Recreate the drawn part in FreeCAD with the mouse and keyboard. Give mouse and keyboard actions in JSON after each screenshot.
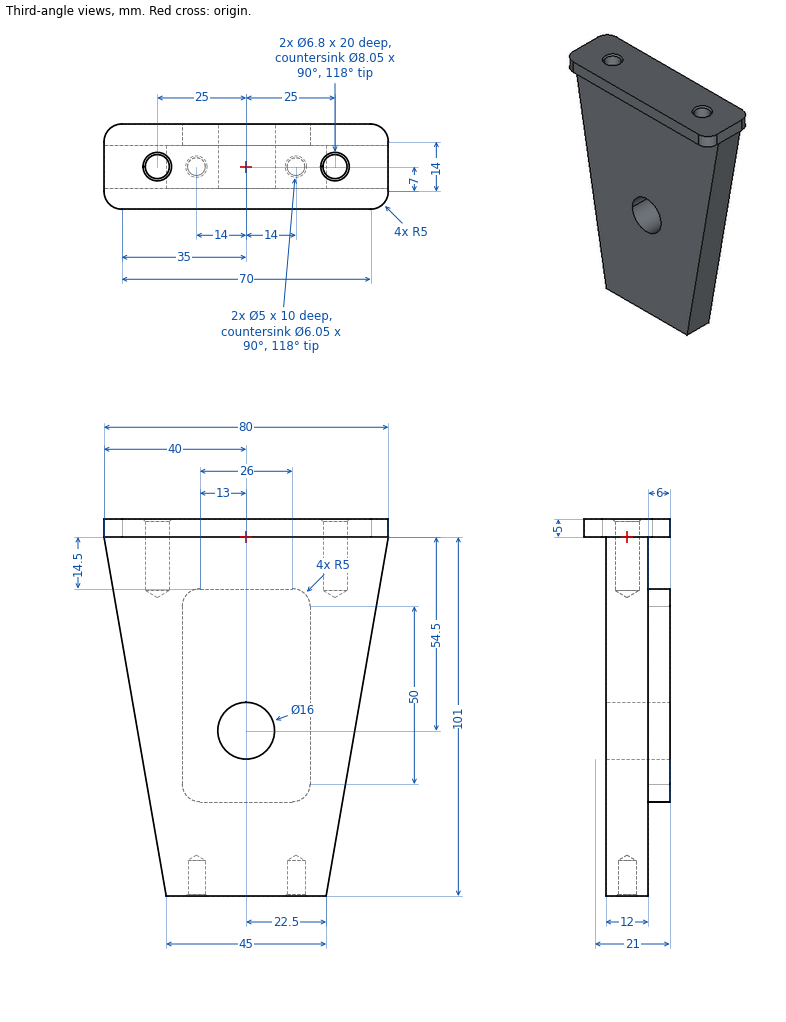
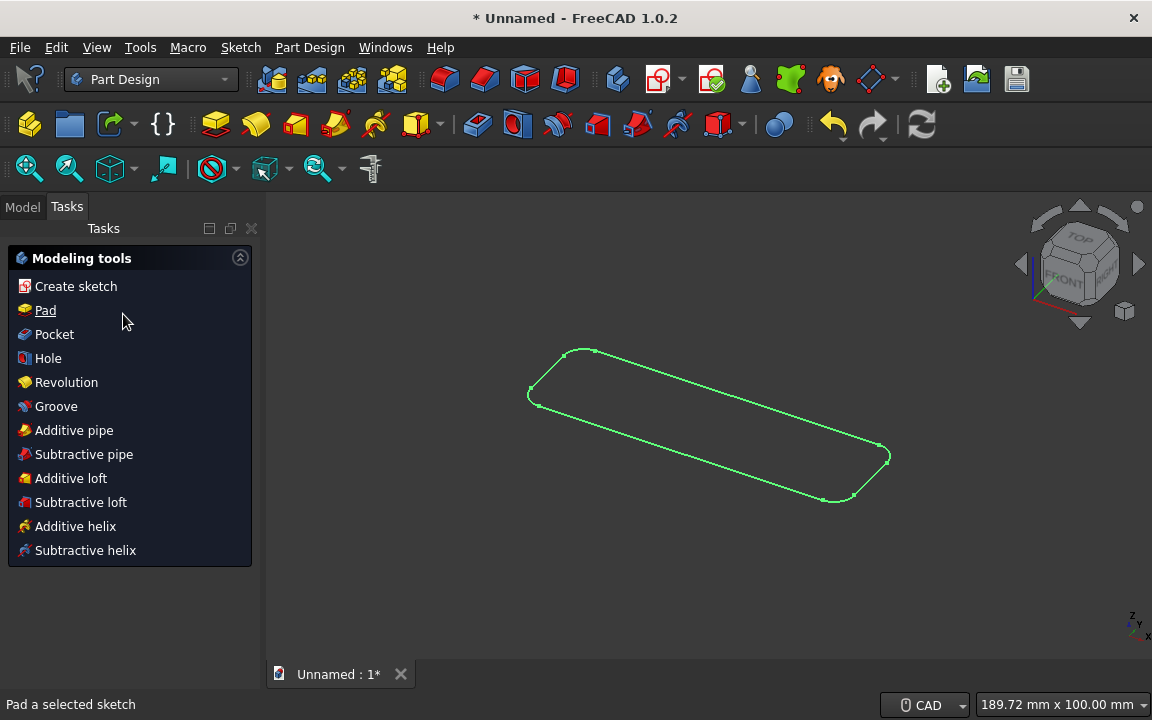
{"action": "left_click", "coordinate": [216, 124]}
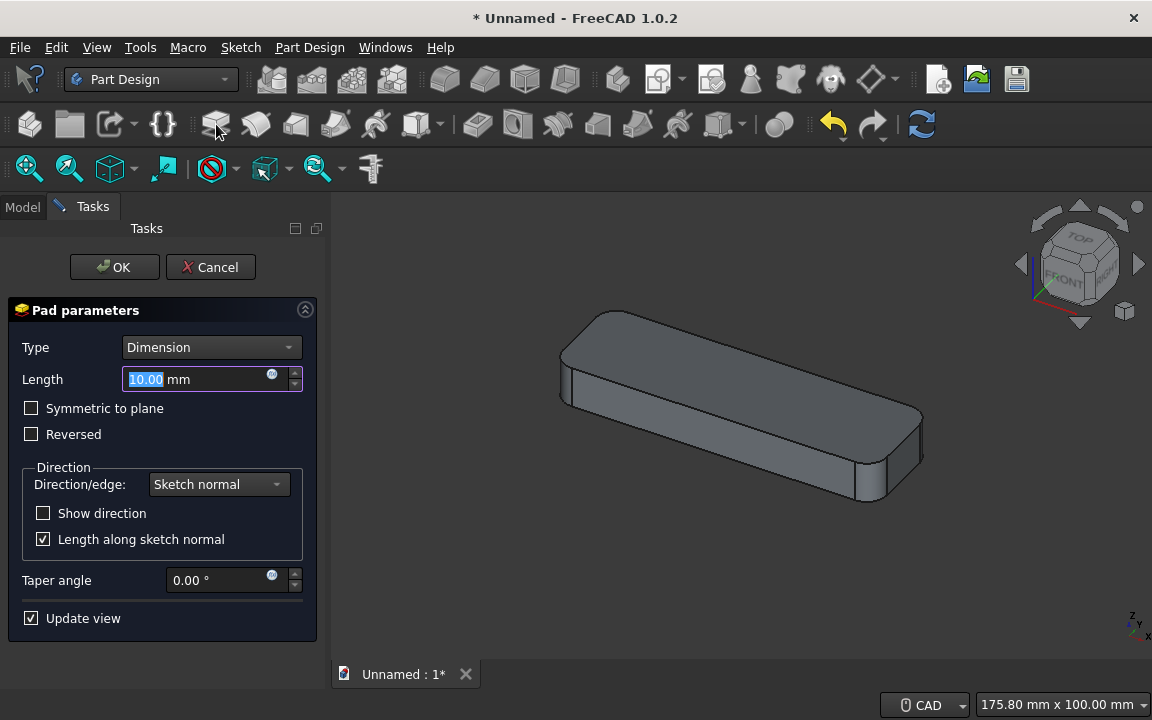
{"action": "type", "text": "5"}
{"action": "key", "text": "Tab"}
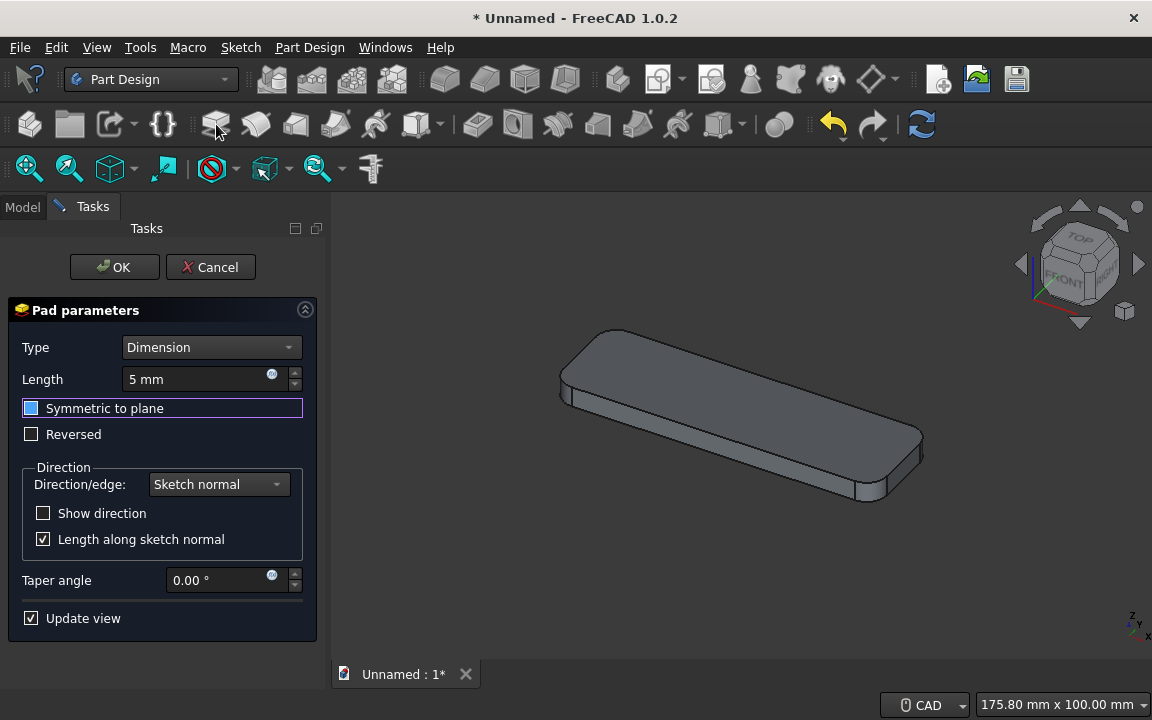
{"action": "left_click", "coordinate": [115, 267]}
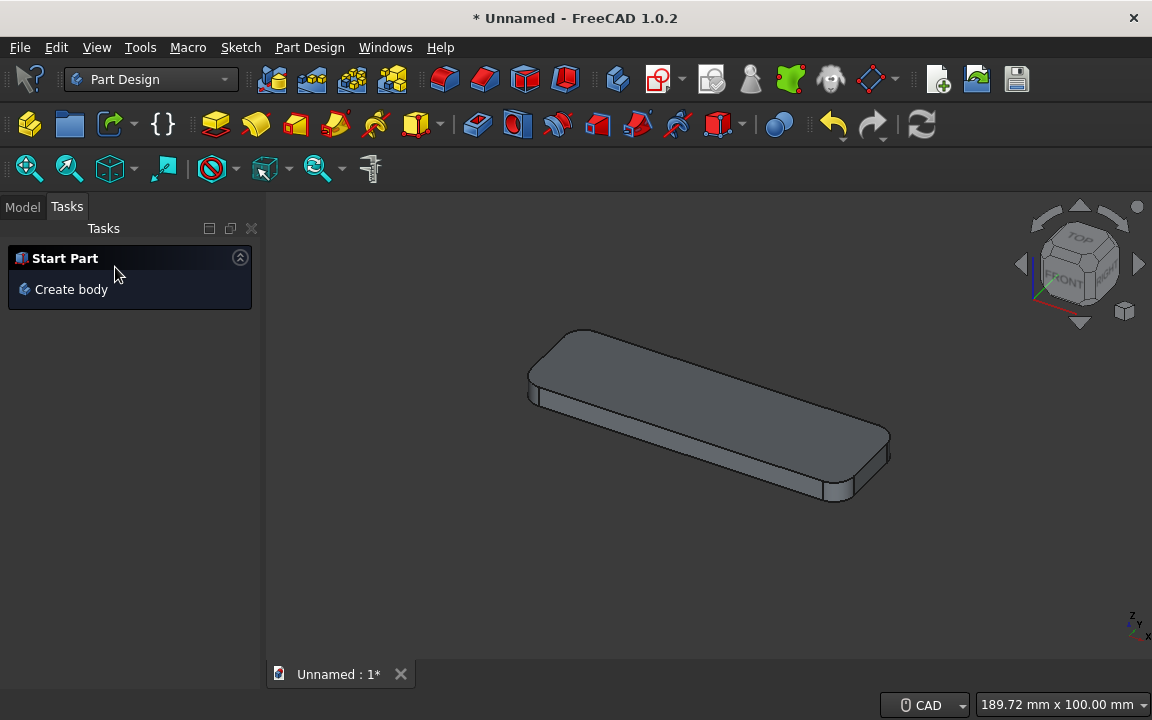
{"action": "left_click", "coordinate": [30, 170]}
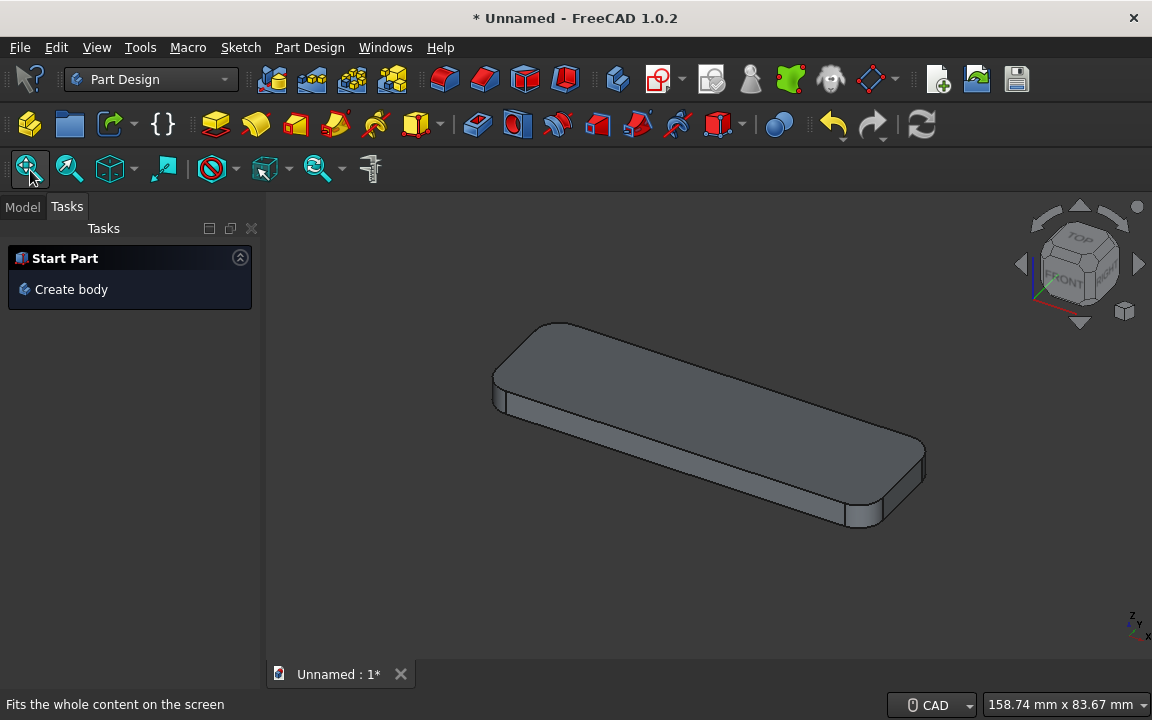
{"action": "left_click", "coordinate": [658, 80]}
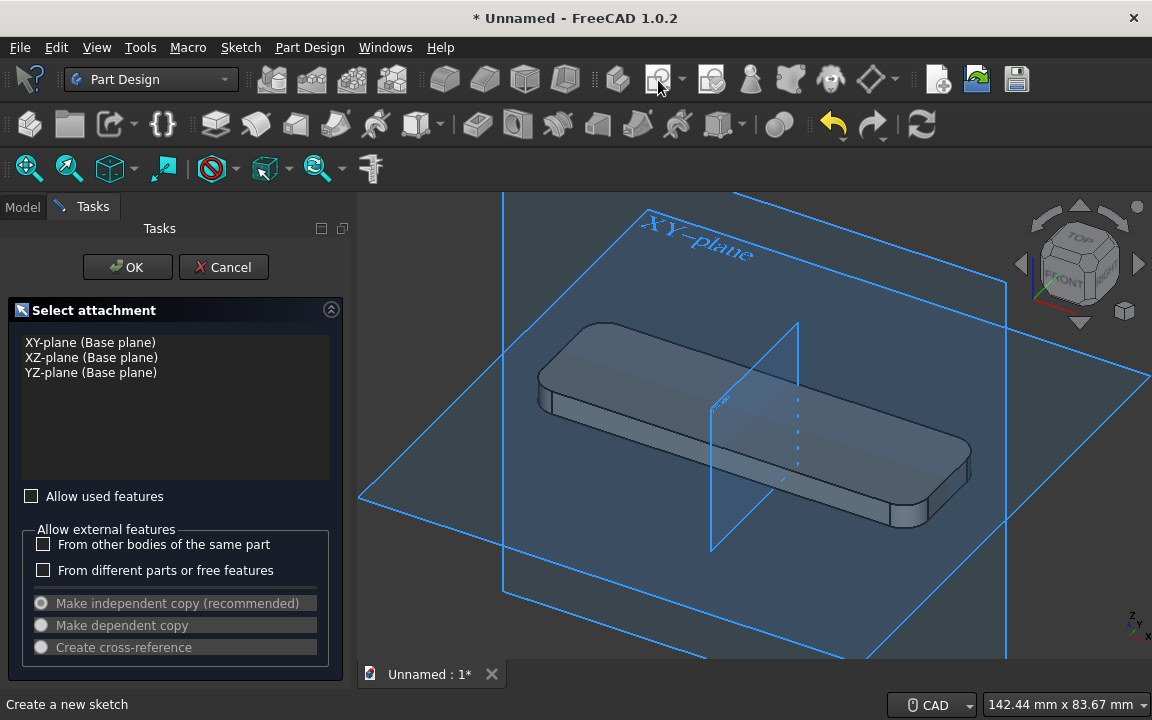
{"action": "left_click", "coordinate": [82, 358]}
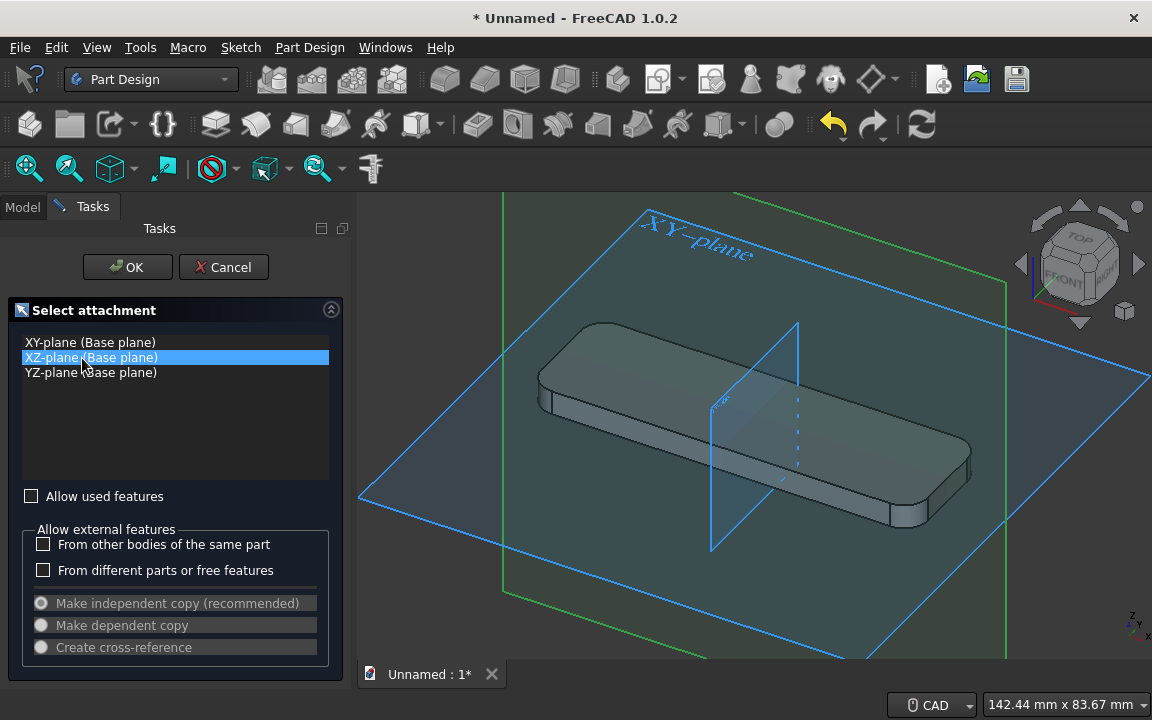
{"action": "left_click", "coordinate": [128, 267]}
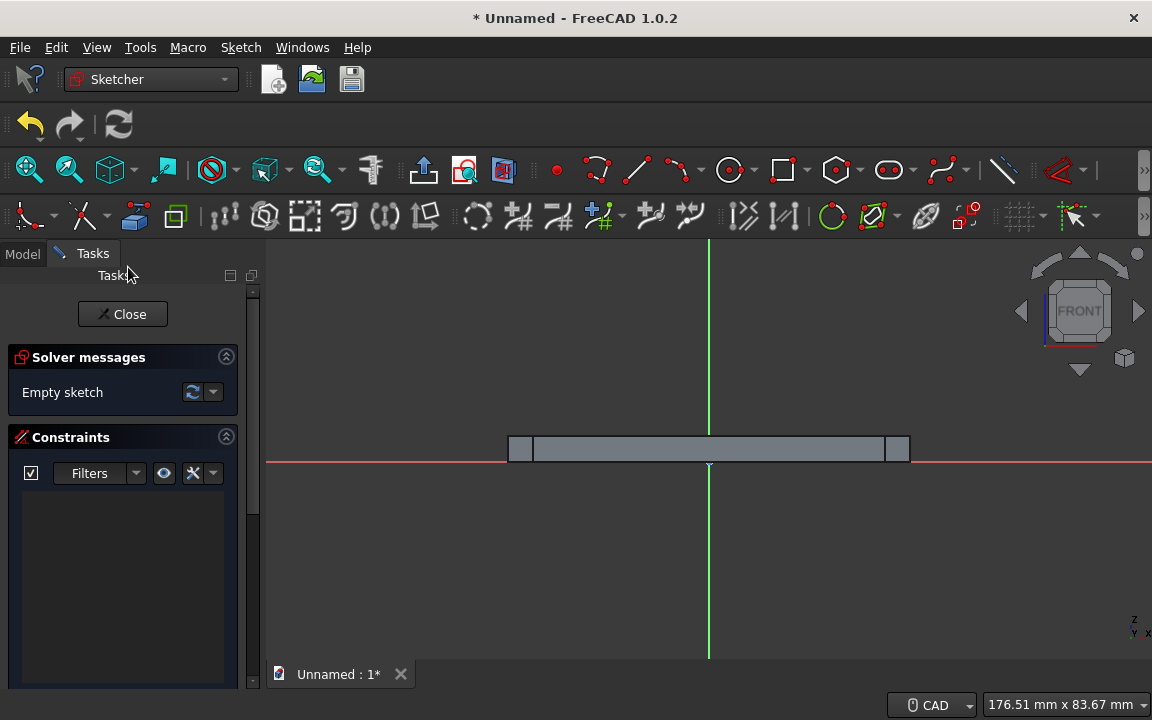
{"action": "left_click", "coordinate": [504, 170]}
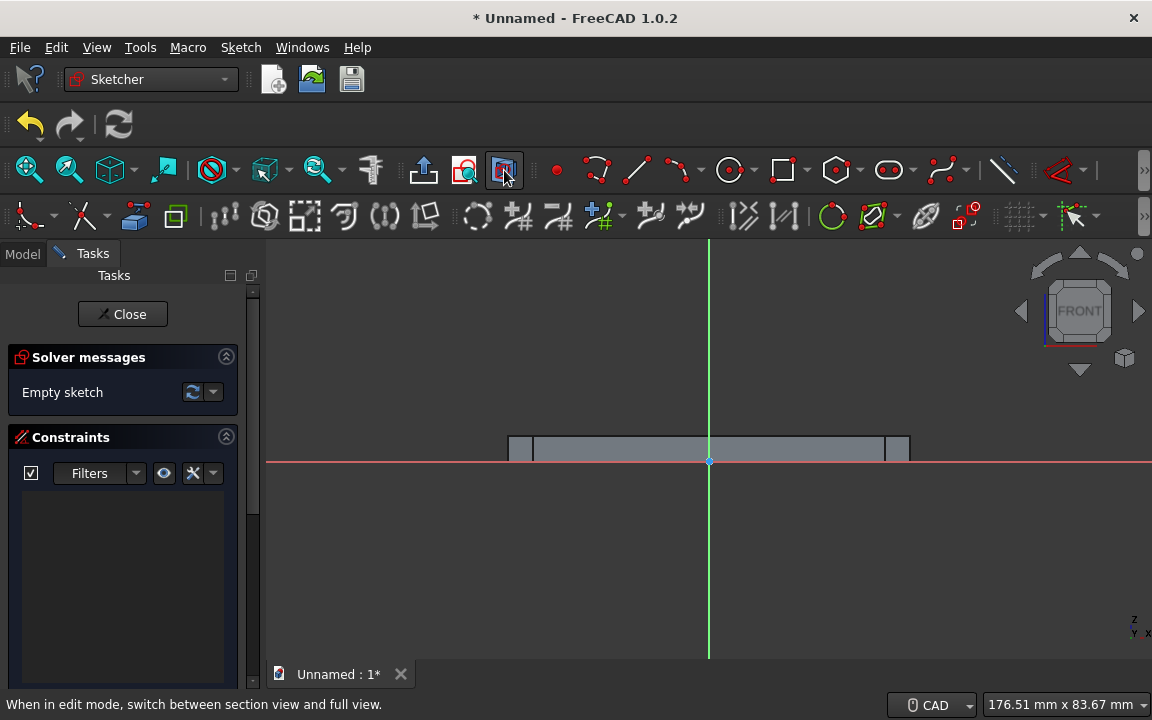
{"action": "scroll", "coordinate": [585, 267], "scroll_direction": "down", "scroll_amount": 4}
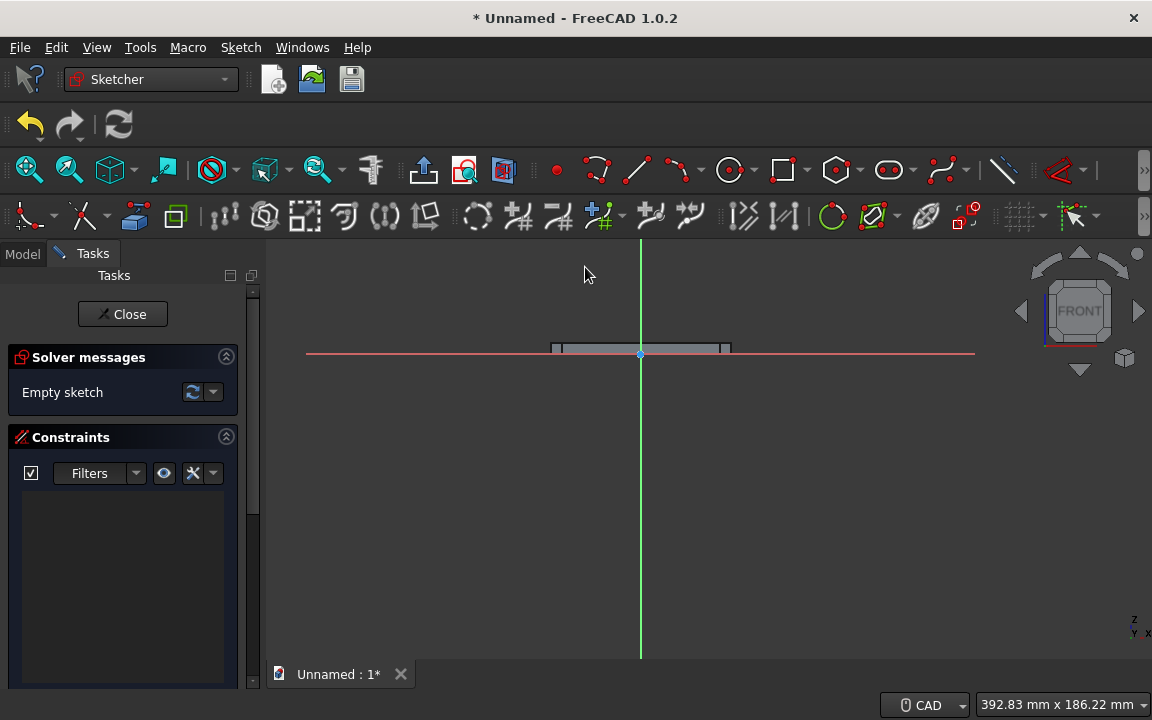
{"action": "left_click", "coordinate": [598, 170]}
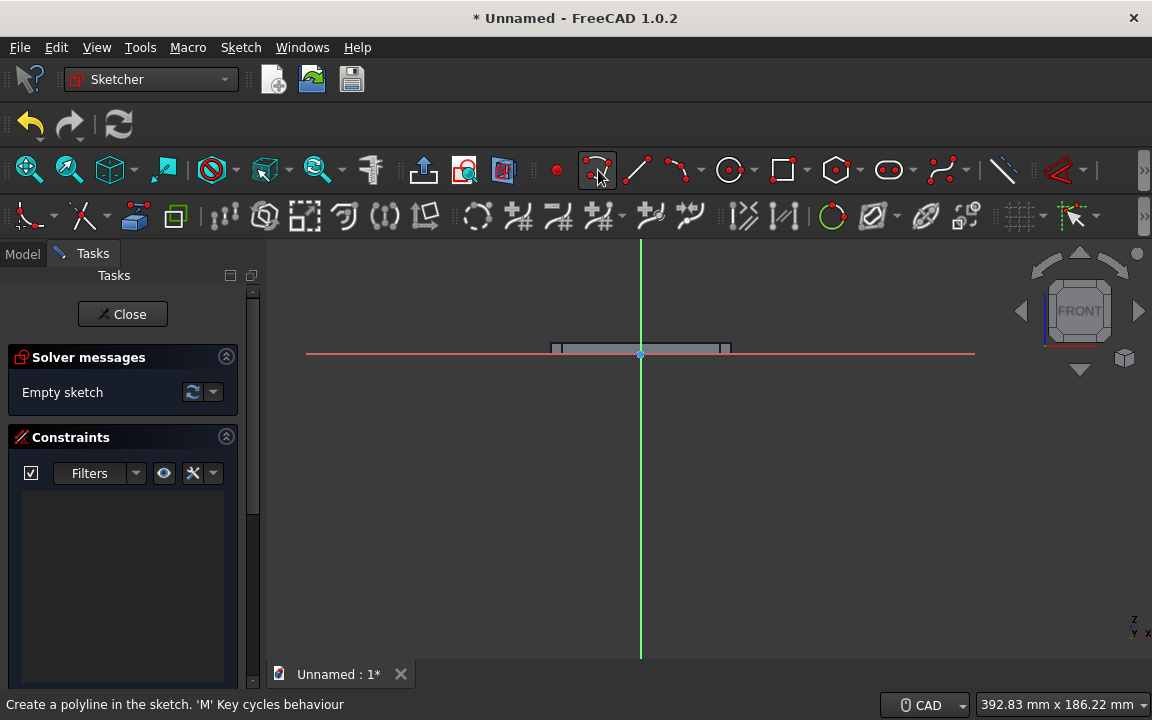
{"action": "left_click", "coordinate": [551, 354]}
{"action": "left_click", "coordinate": [731, 363]}
{"action": "left_click", "coordinate": [692, 582]}
{"action": "left_click", "coordinate": [590, 582]}
{"action": "left_click", "coordinate": [551, 354]}
{"action": "key", "text": "Escape"}
{"action": "key", "text": "Escape"}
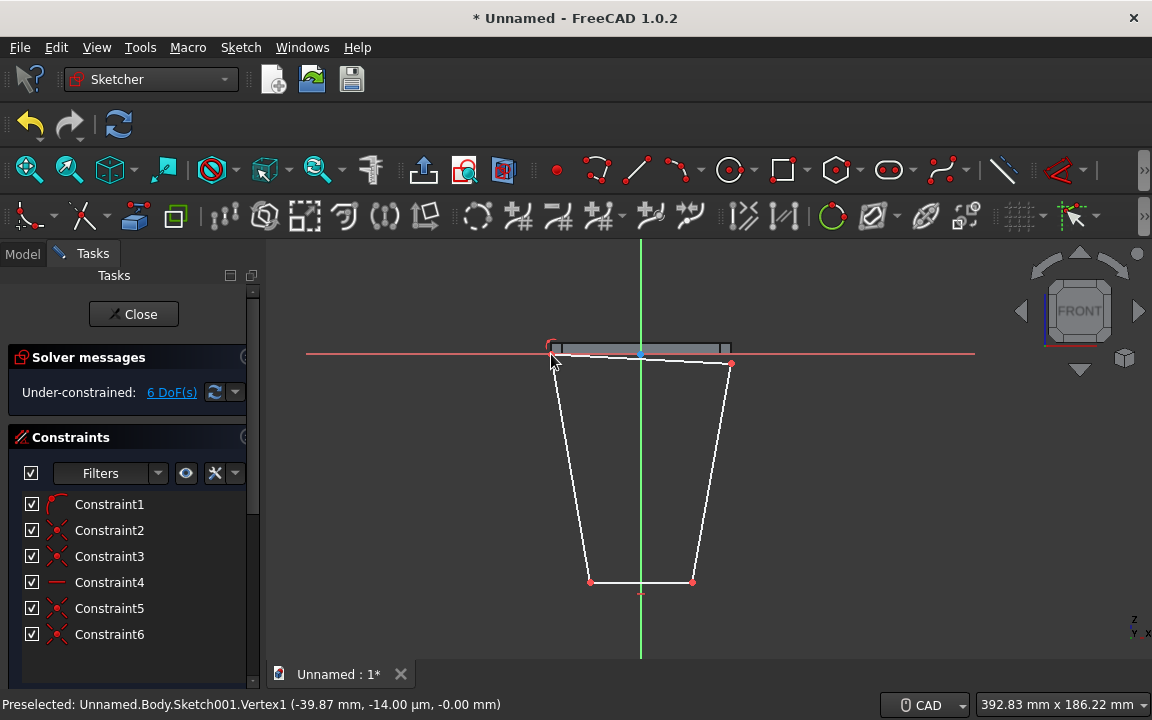
{"action": "left_click", "coordinate": [605, 357]}